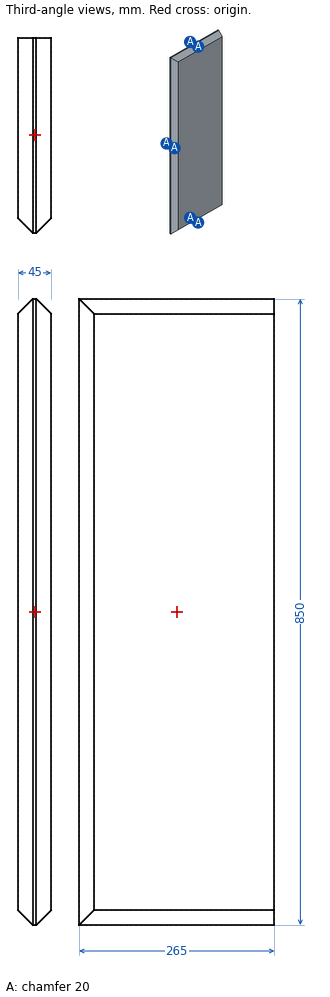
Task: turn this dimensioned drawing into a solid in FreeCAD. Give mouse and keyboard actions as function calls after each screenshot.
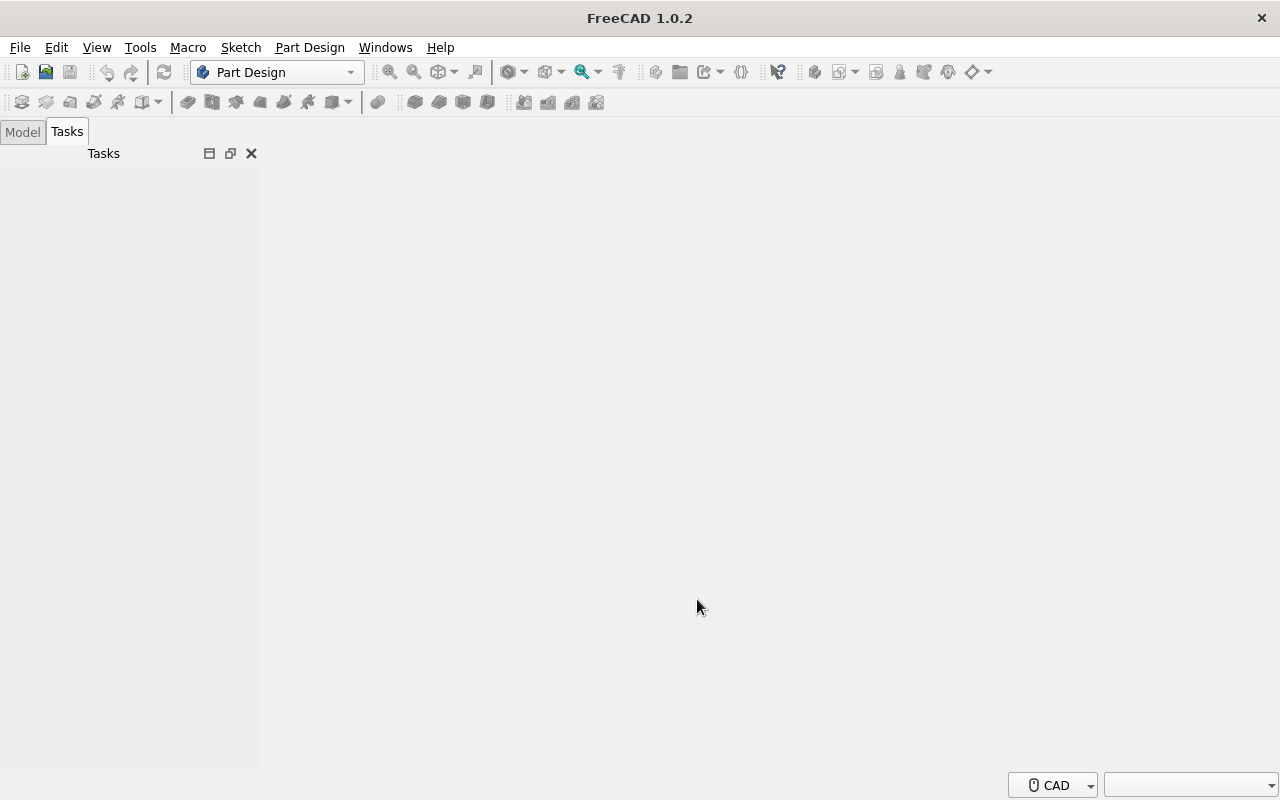
key(ctrl+n)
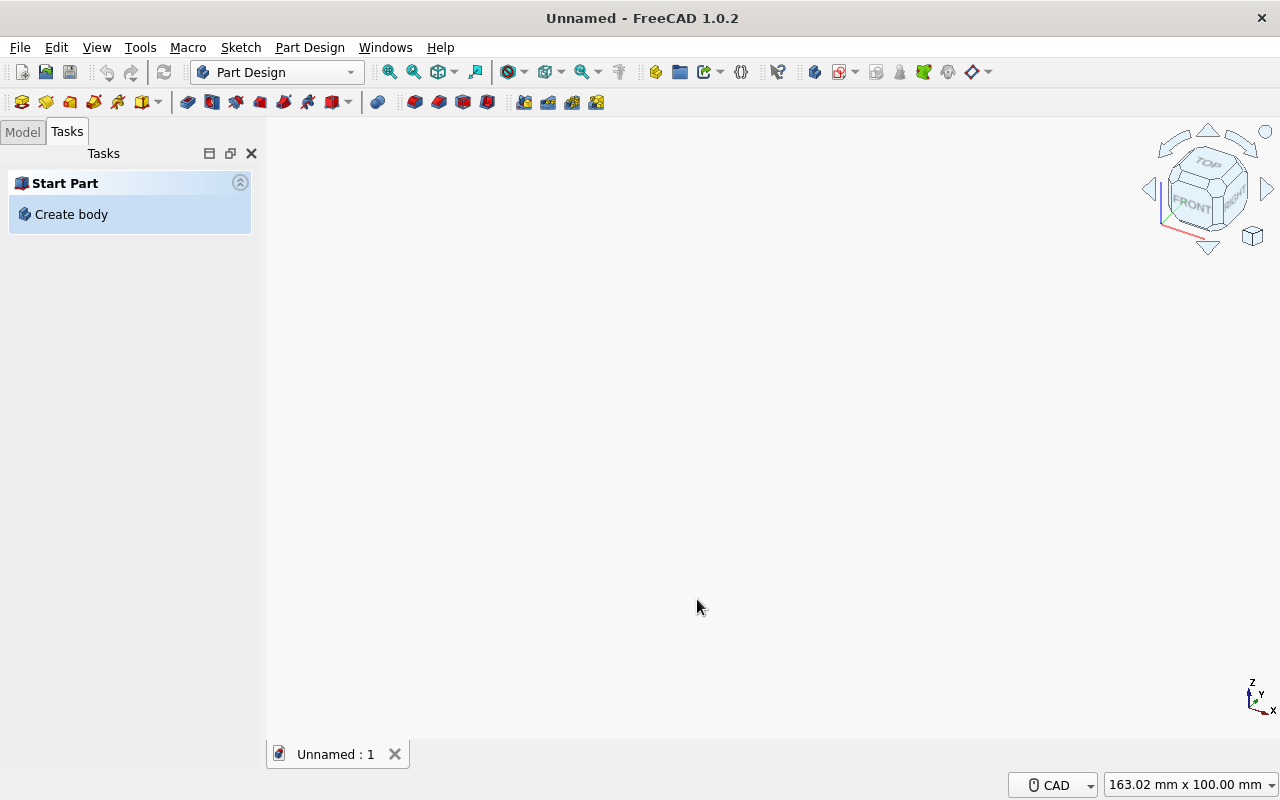
click(840, 72)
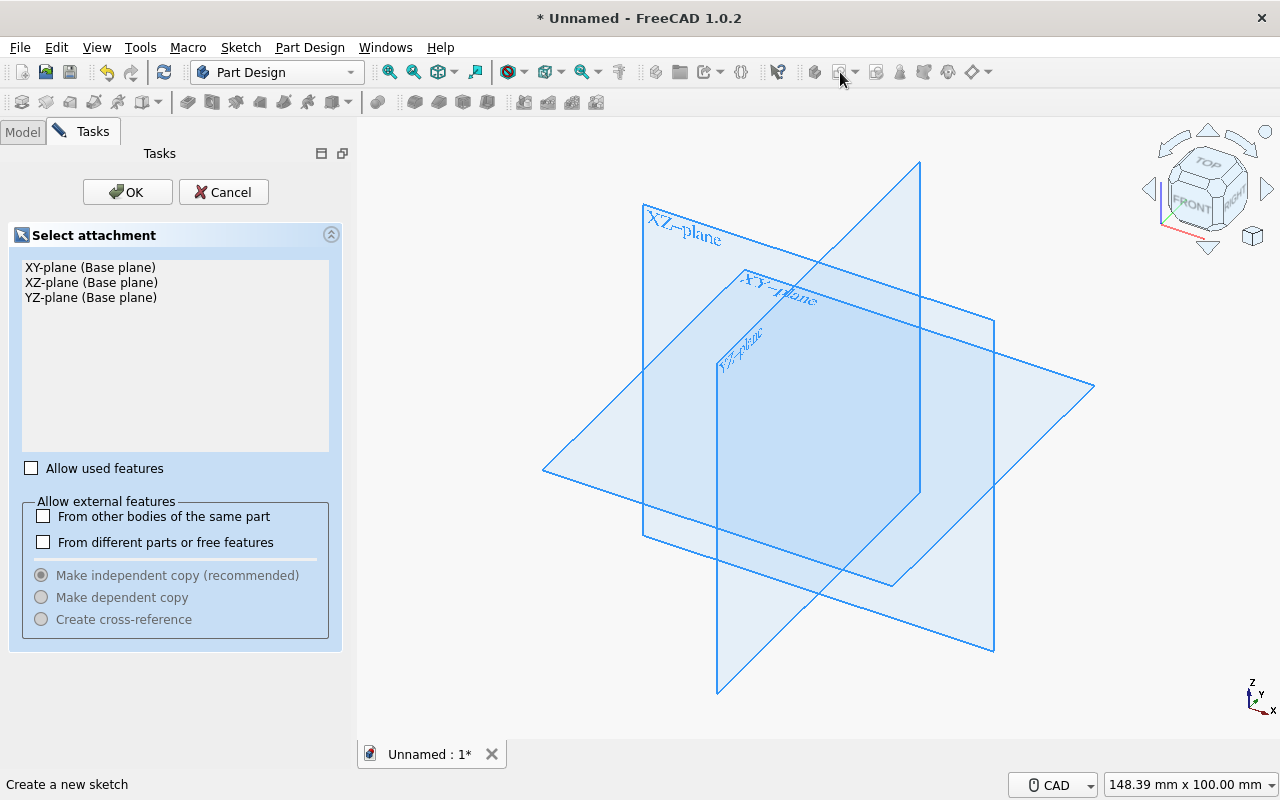
click(82, 298)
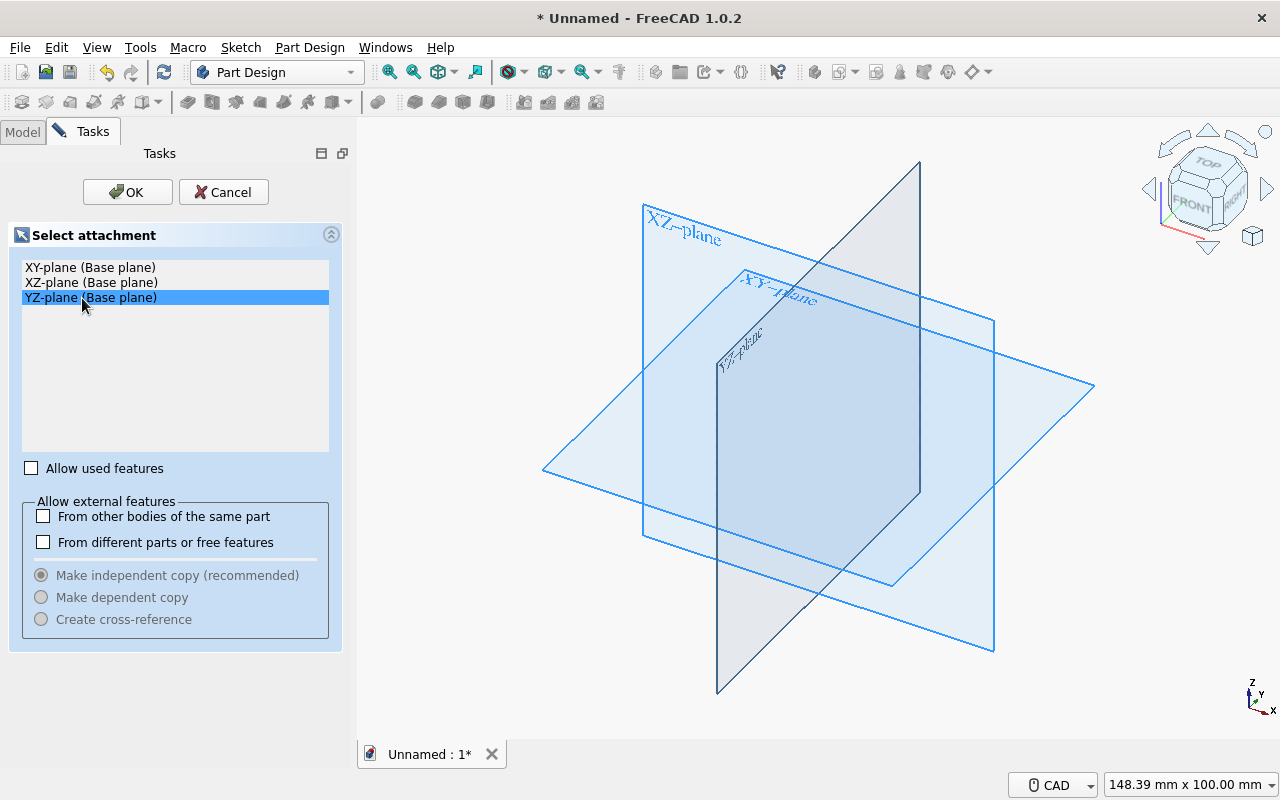
click(128, 192)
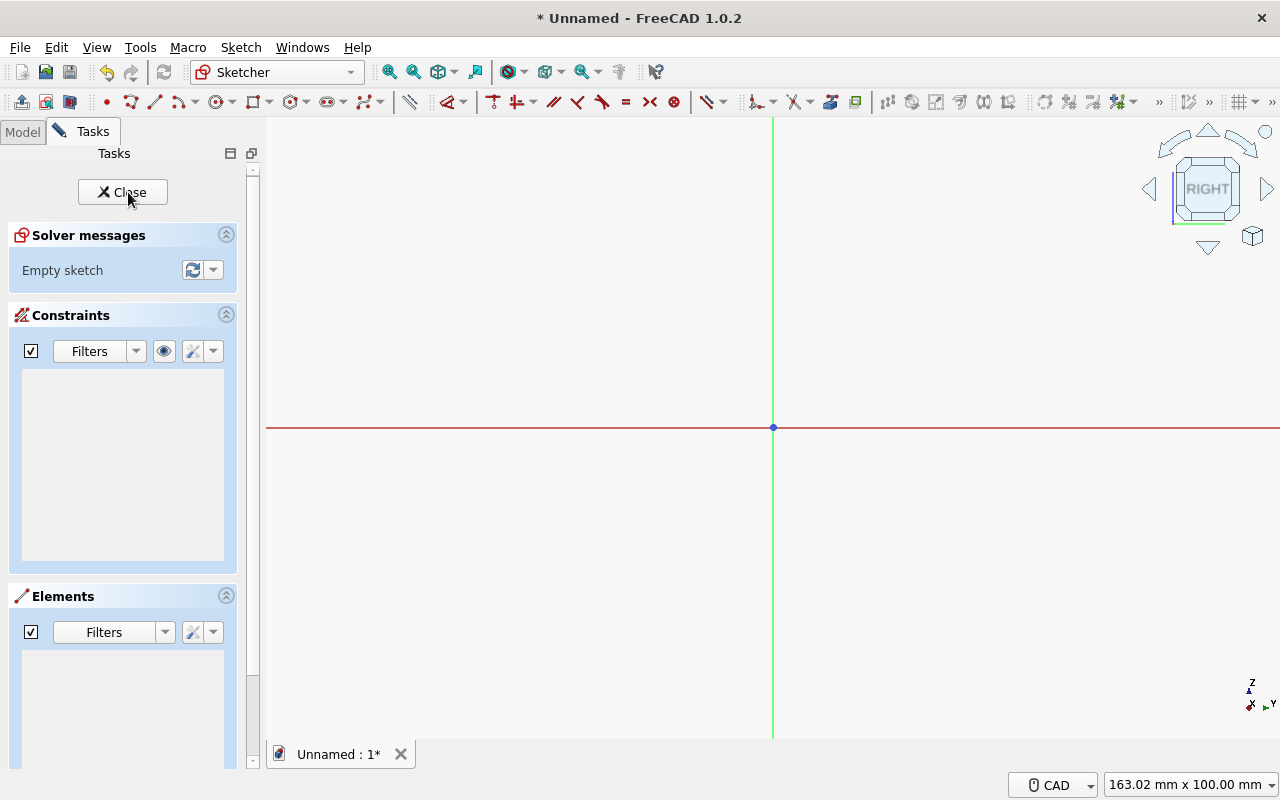
scroll(699, 428, down, 13)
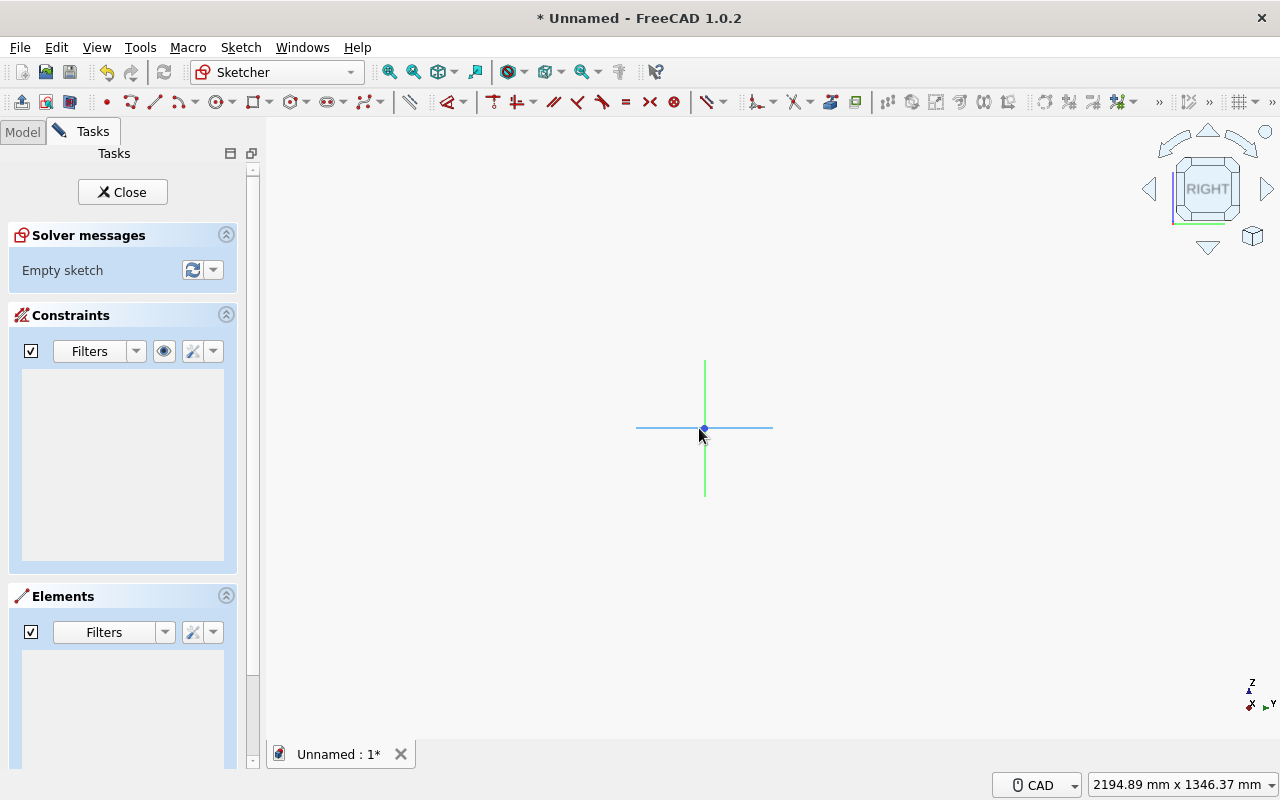
key(g)
key(v)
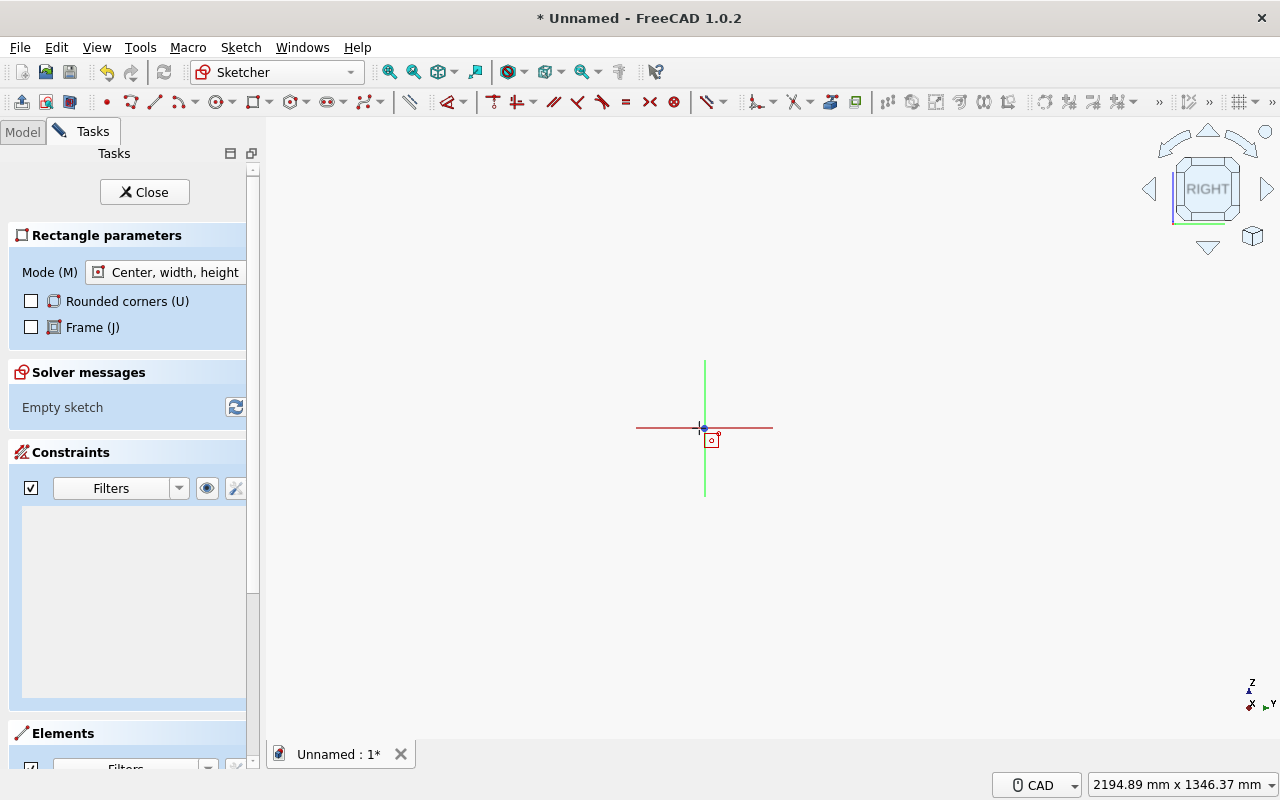
click(705, 428)
move(766, 232)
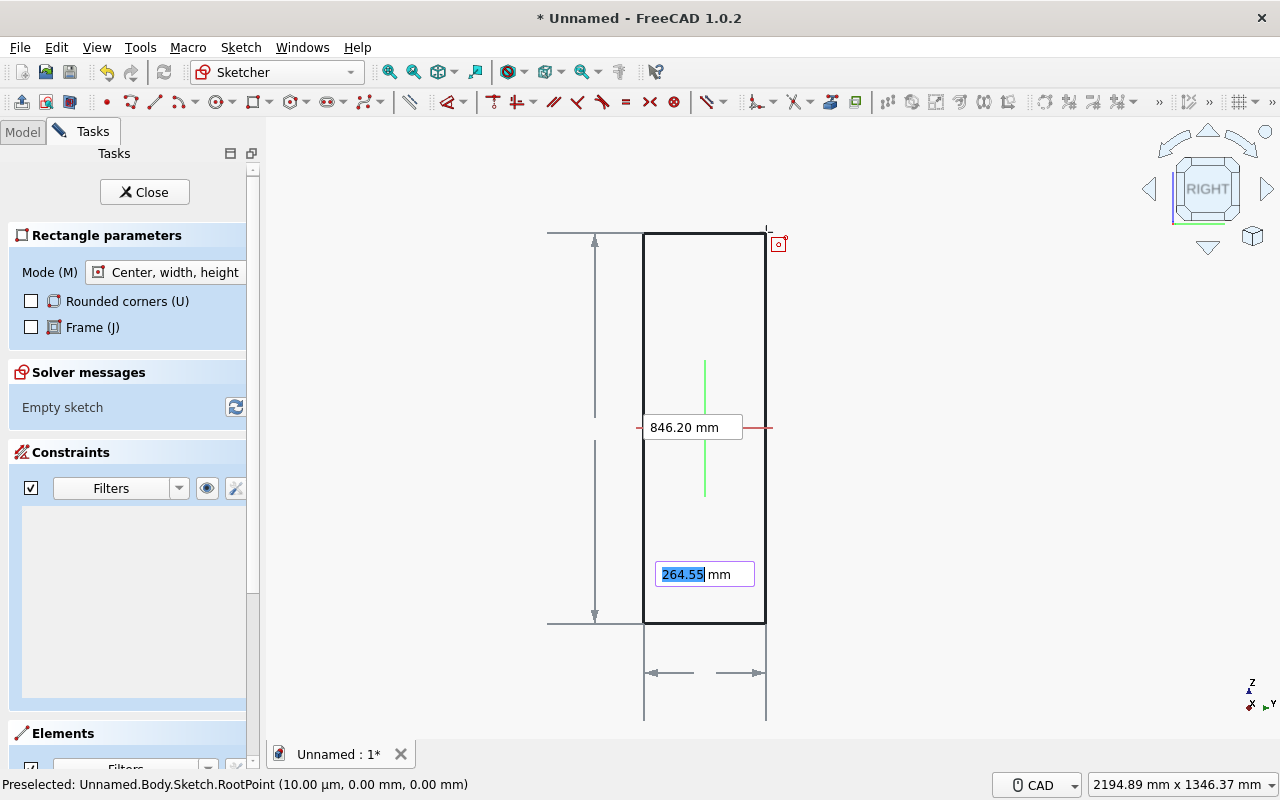
text(265)
key(Tab)
text(850)
key(Return)
key(Escape)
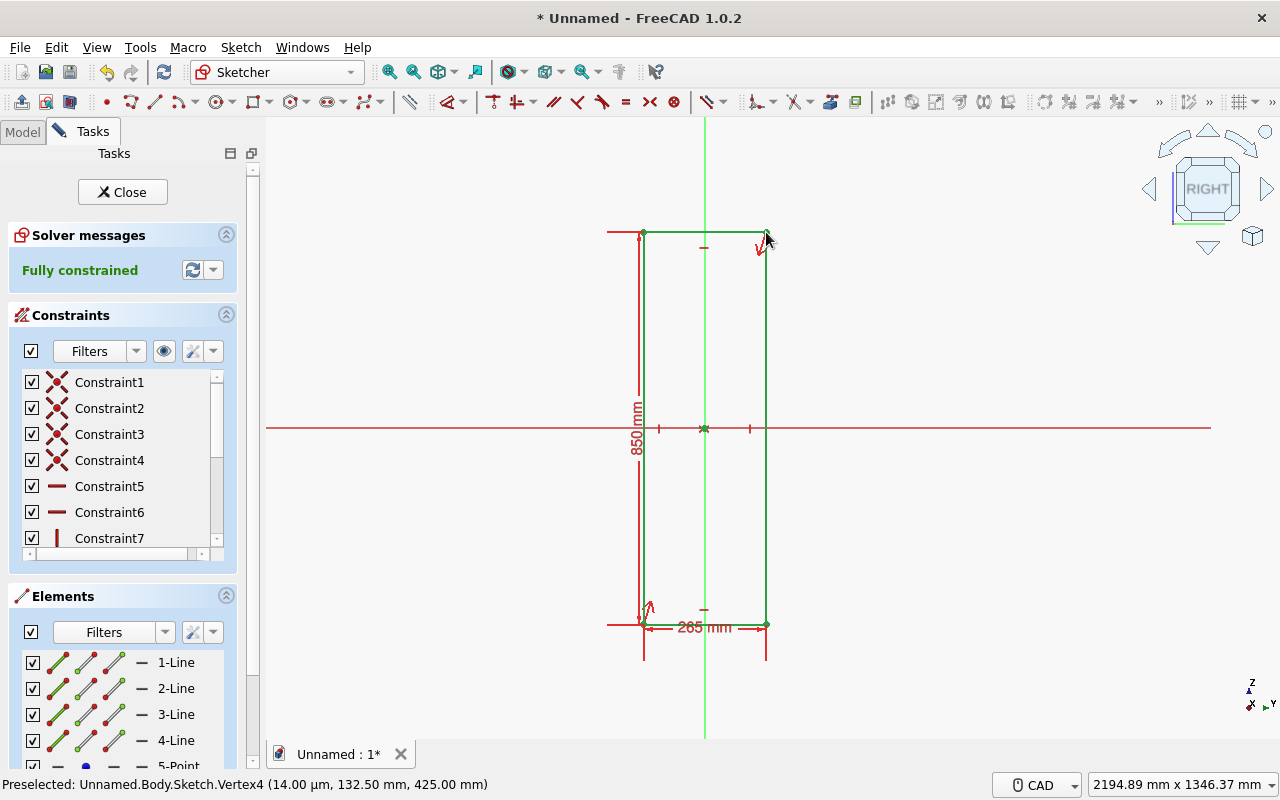
click(123, 192)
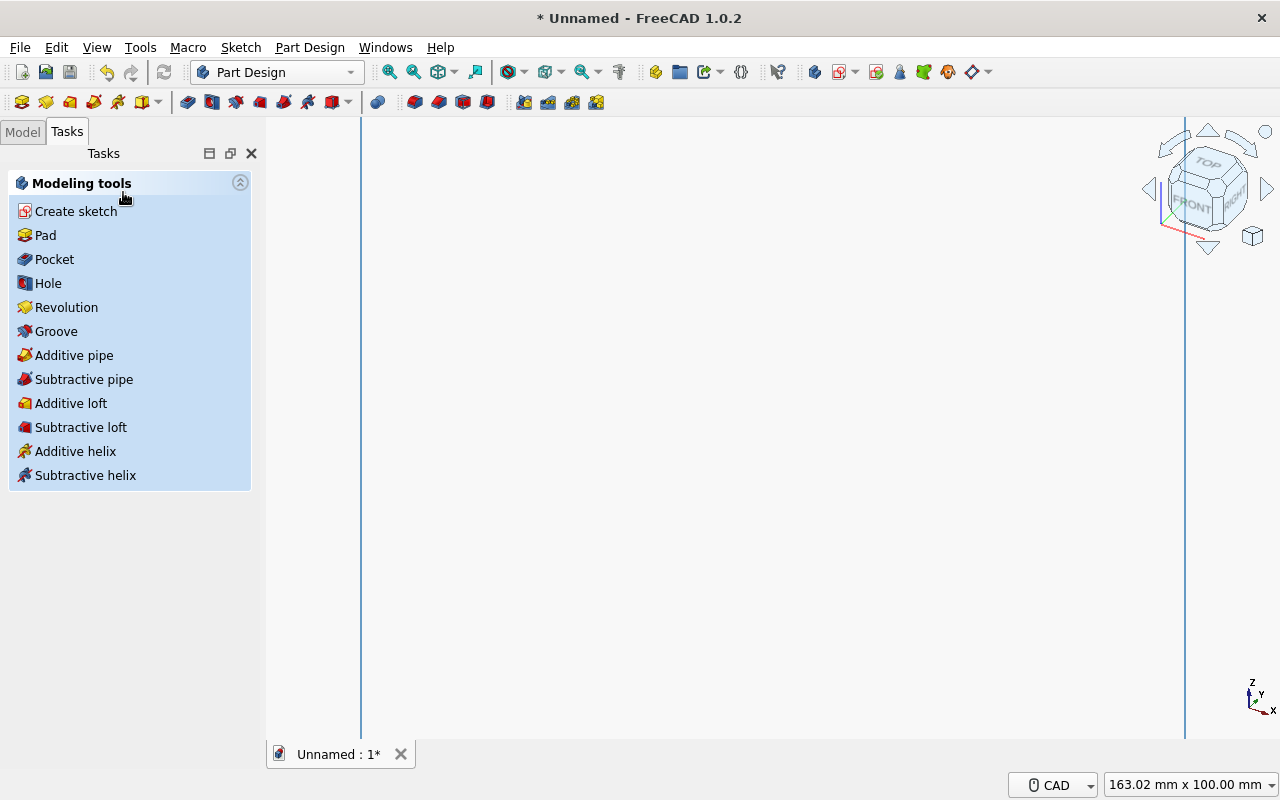
click(22, 102)